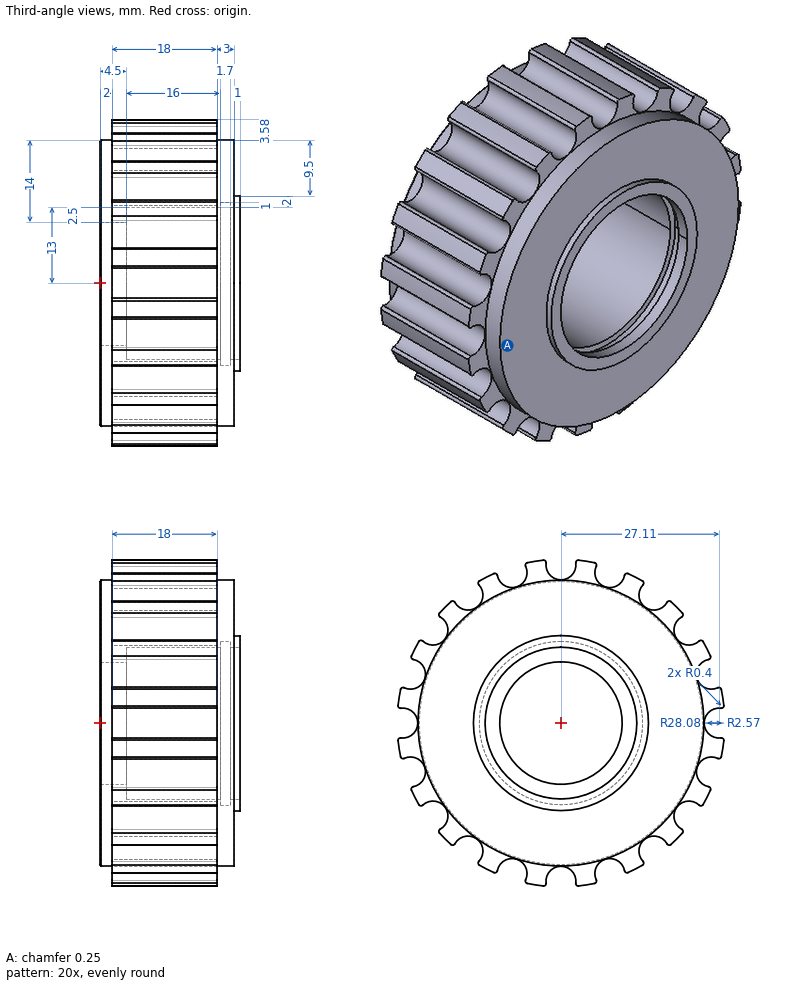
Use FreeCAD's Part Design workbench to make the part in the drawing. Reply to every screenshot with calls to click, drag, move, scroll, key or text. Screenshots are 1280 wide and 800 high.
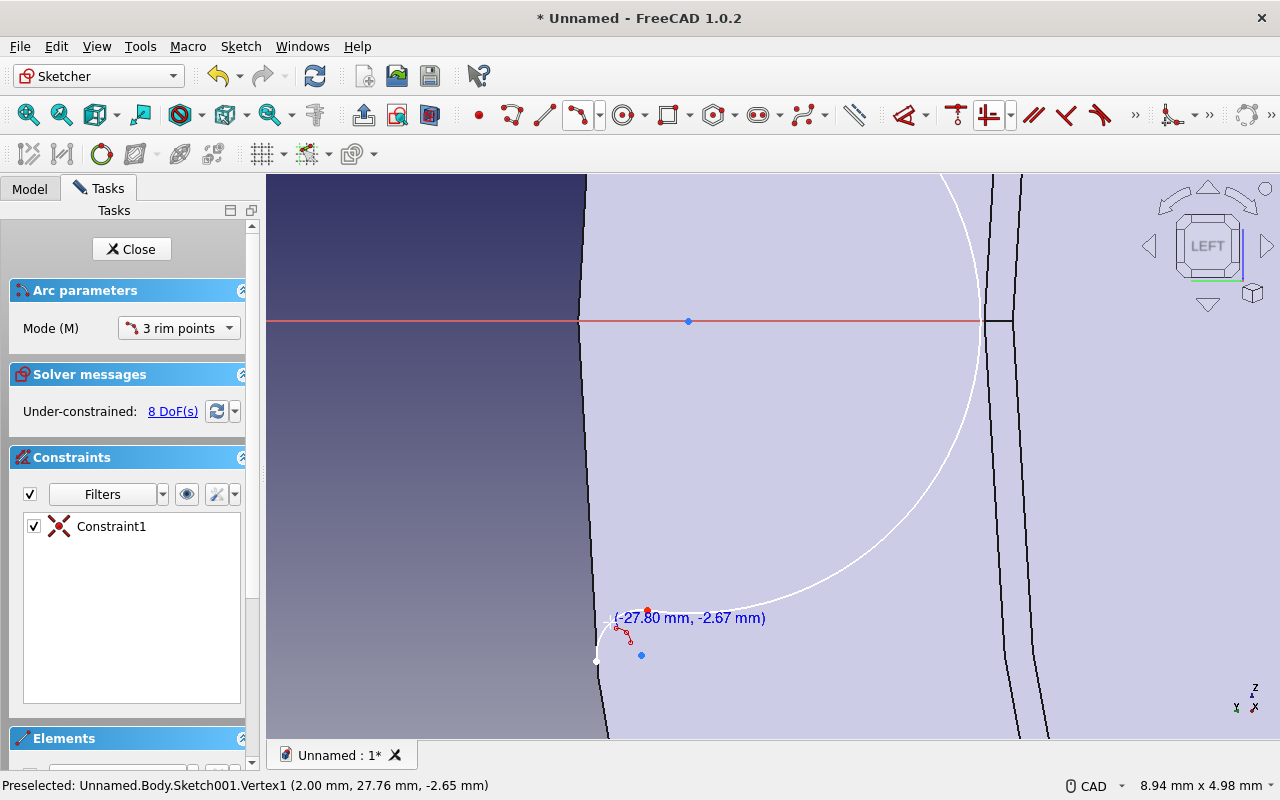
click(597, 661)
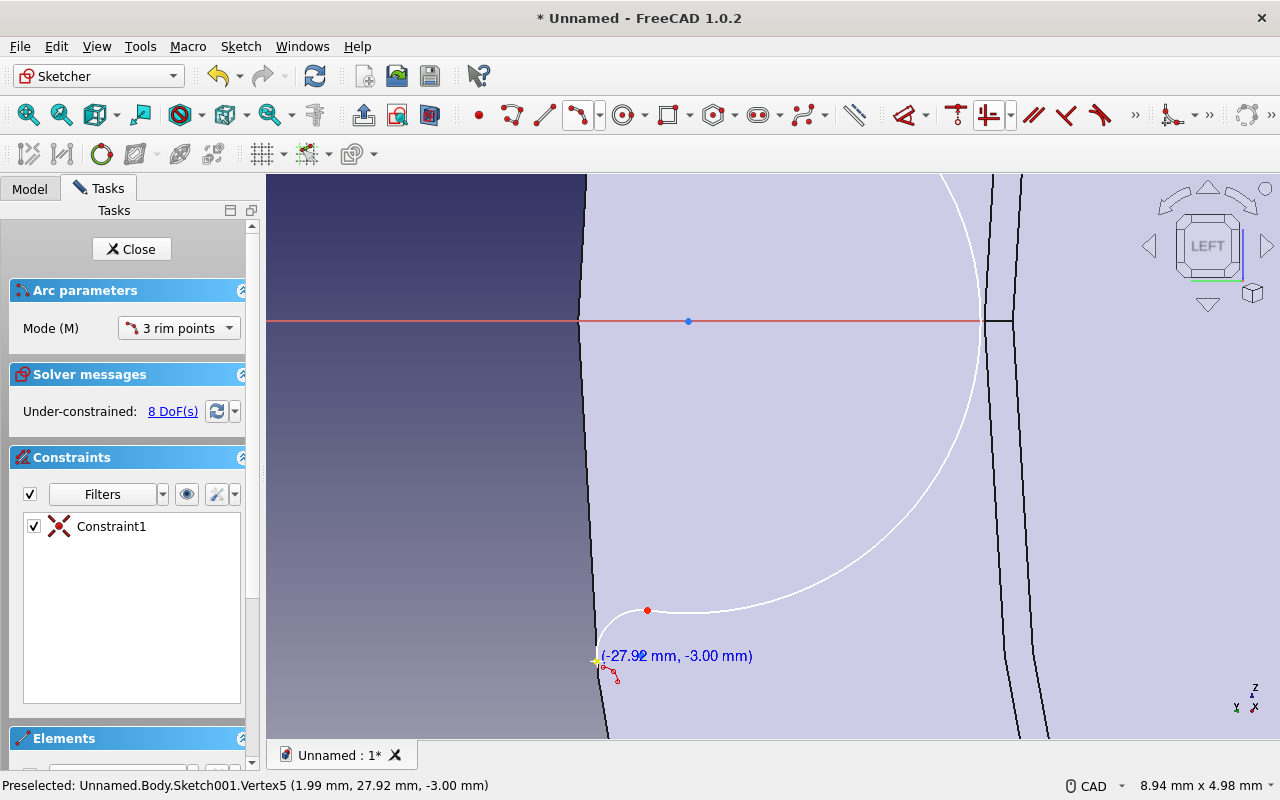
scroll(614, 622, down, 3)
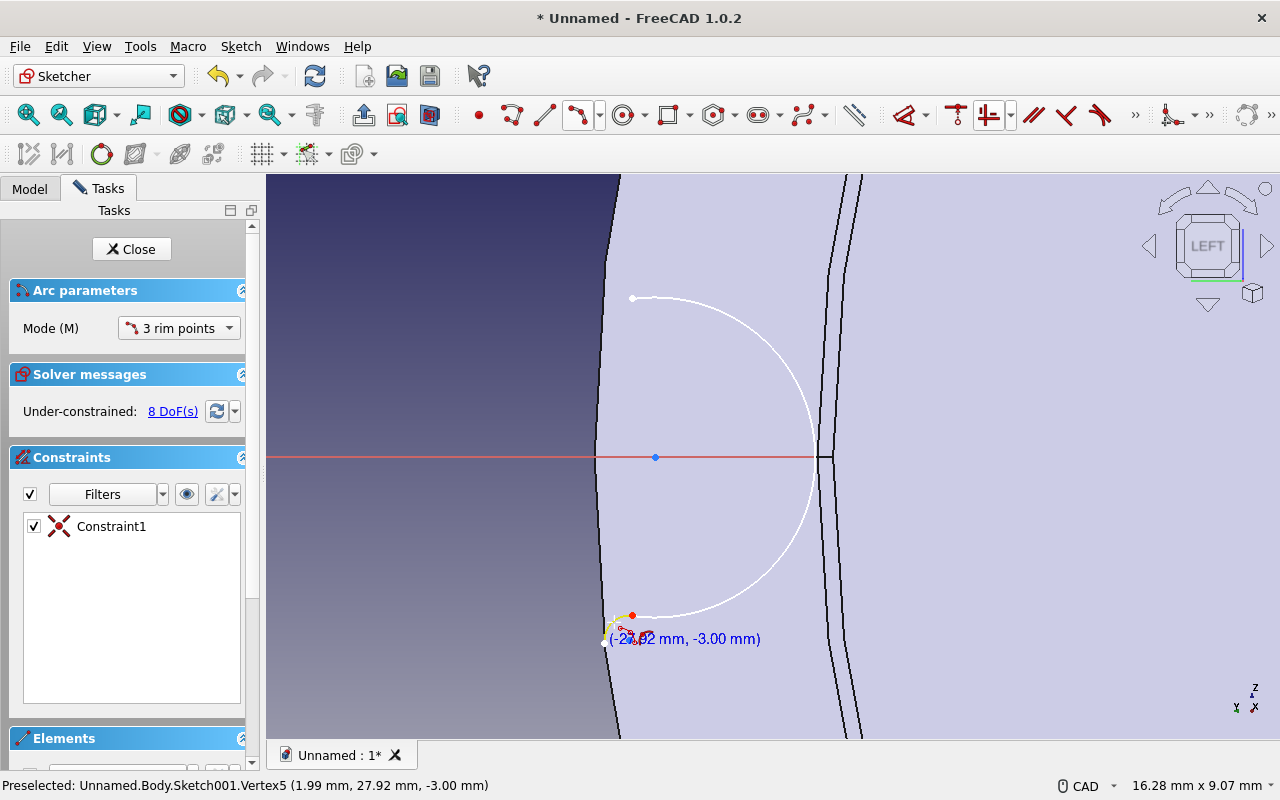
click(604, 271)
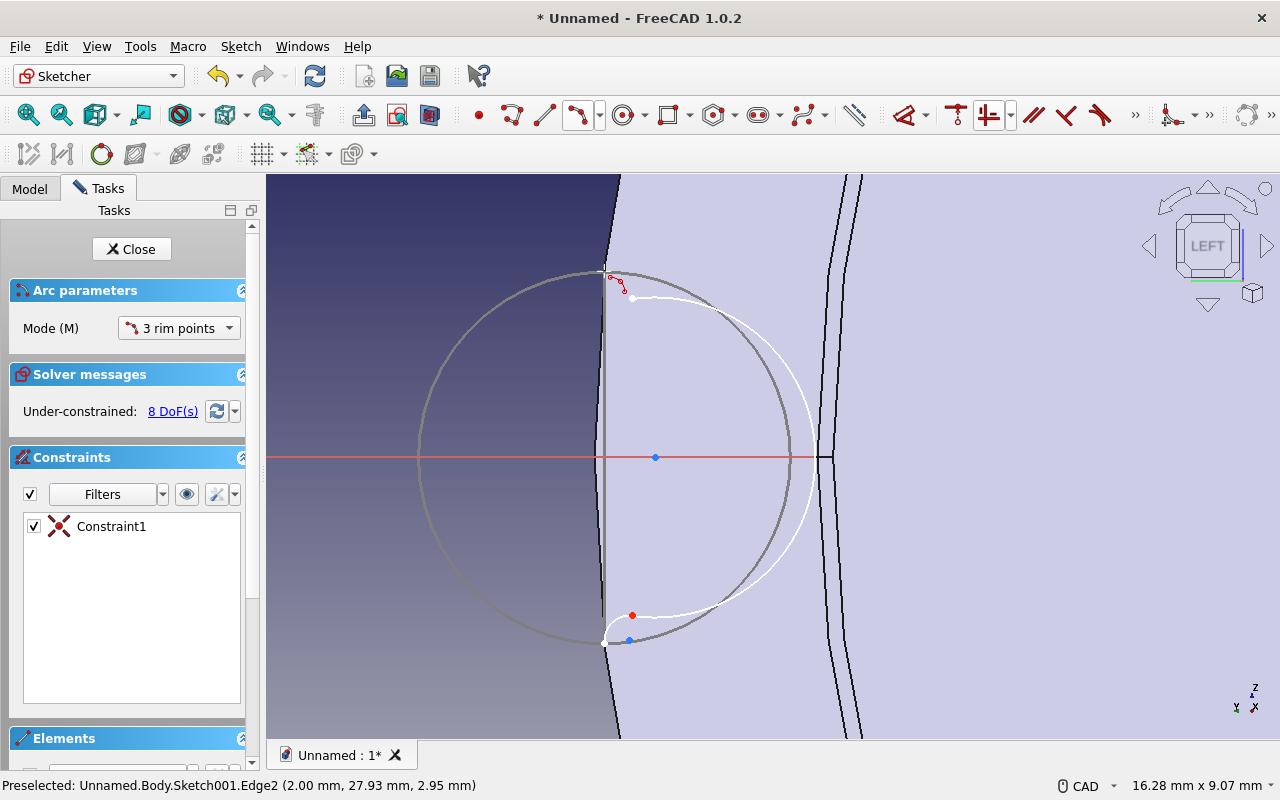
scroll(595, 420, up, 3)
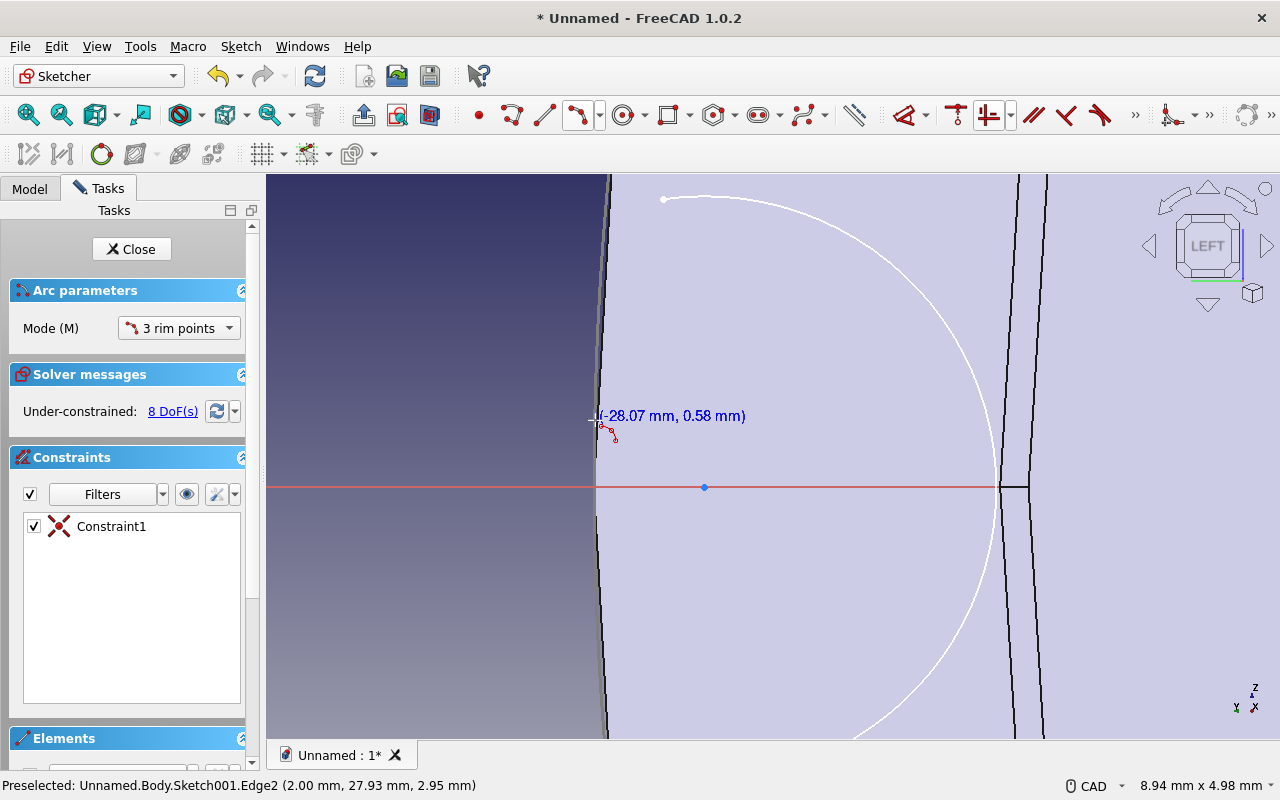
click(595, 419)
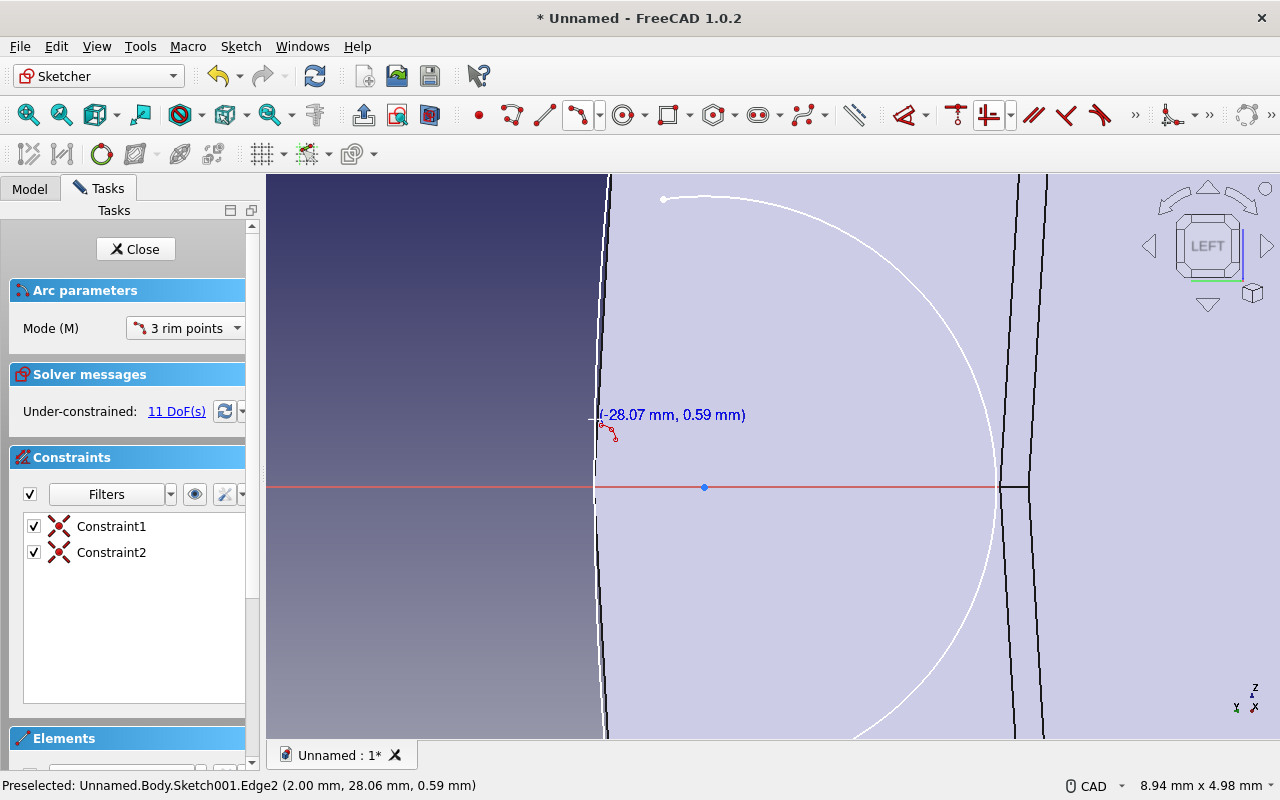
scroll(595, 419, down, 3)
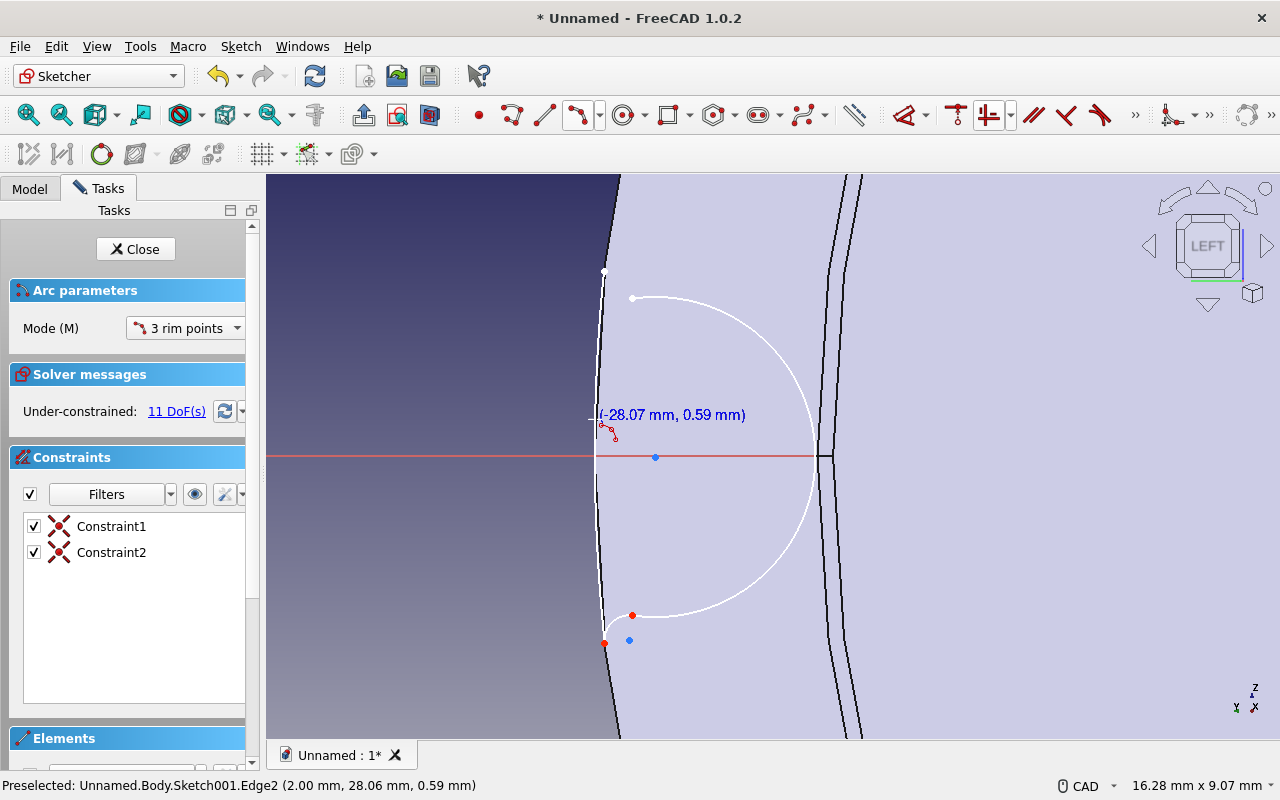
click(604, 272)
click(633, 299)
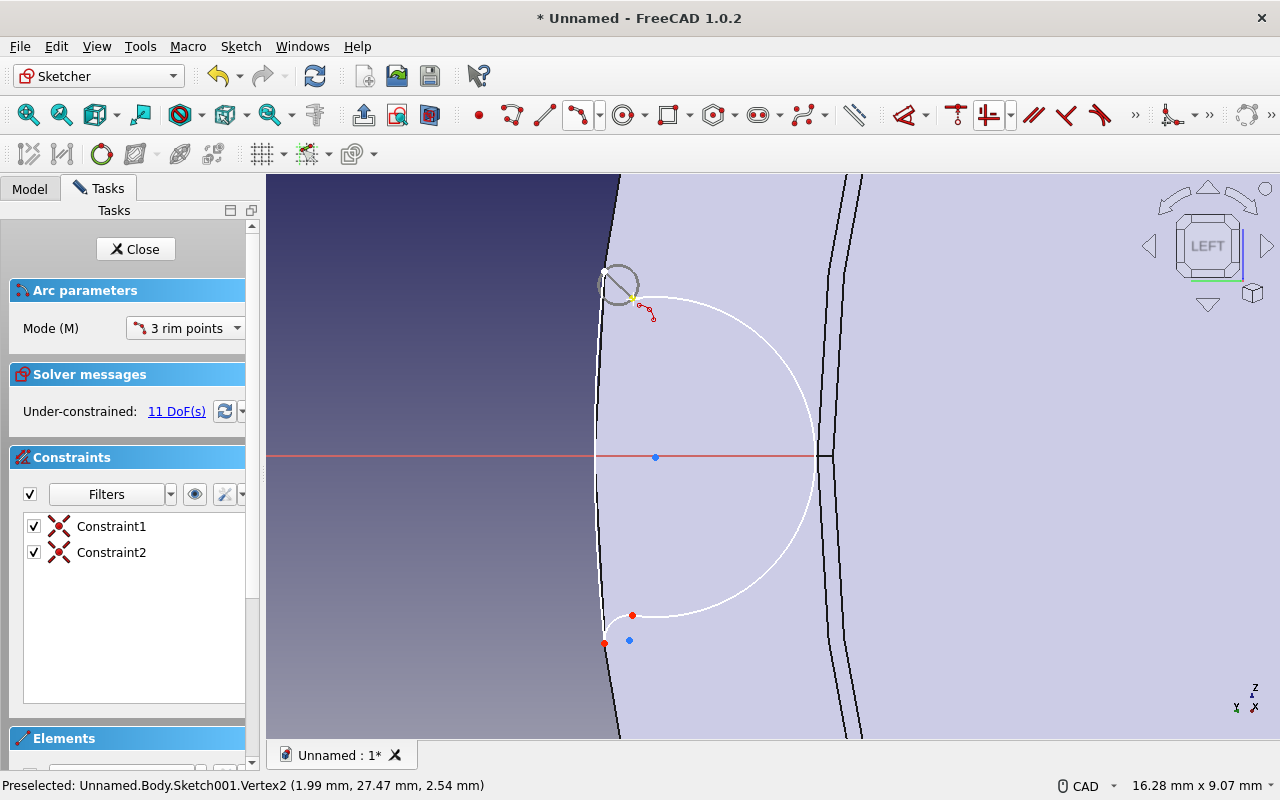
scroll(612, 291, up, 3)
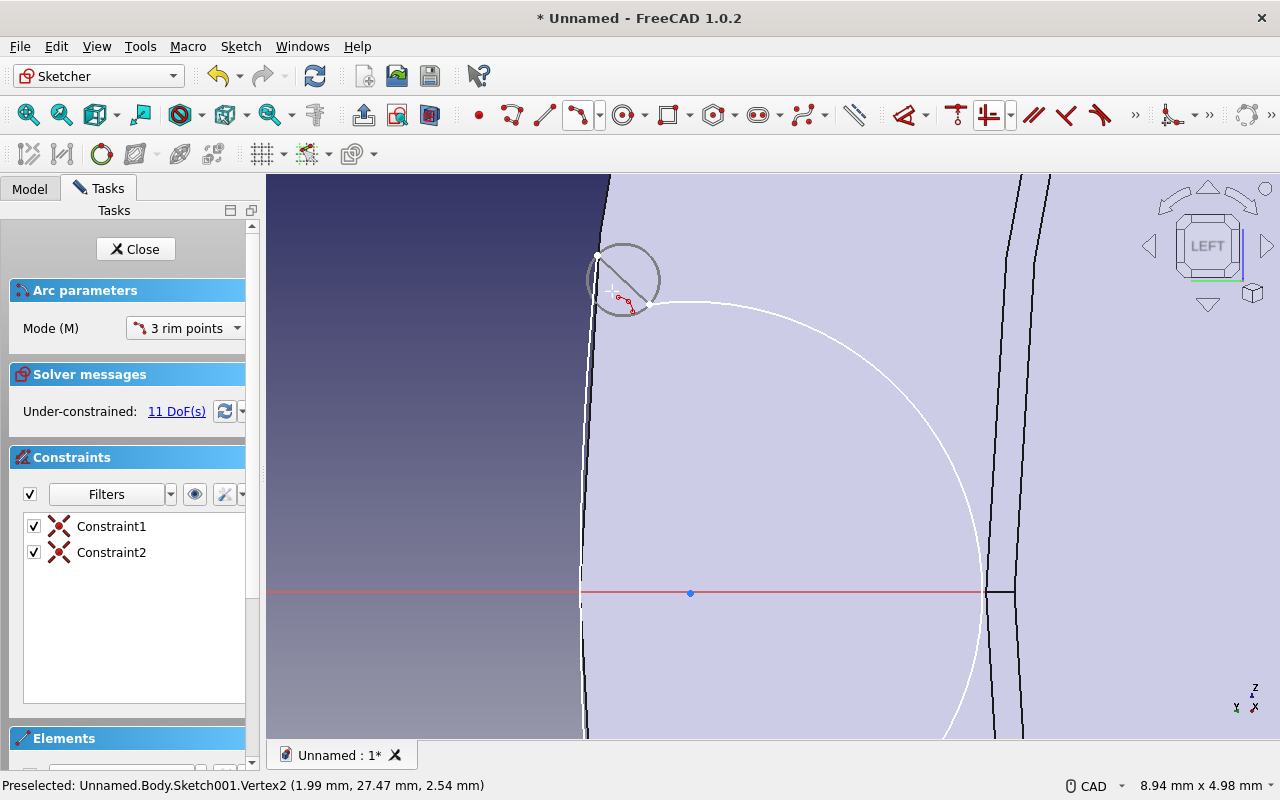
click(612, 291)
key(Escape)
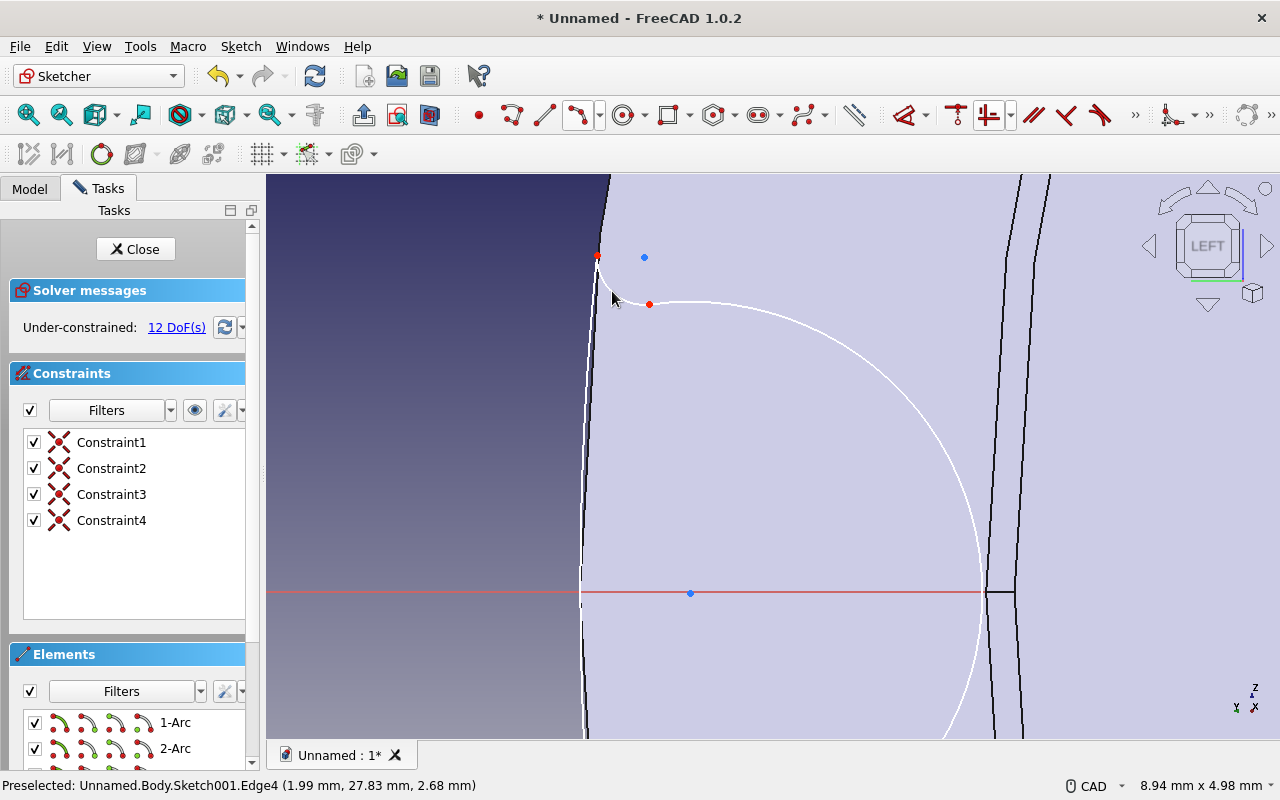
click(917, 409)